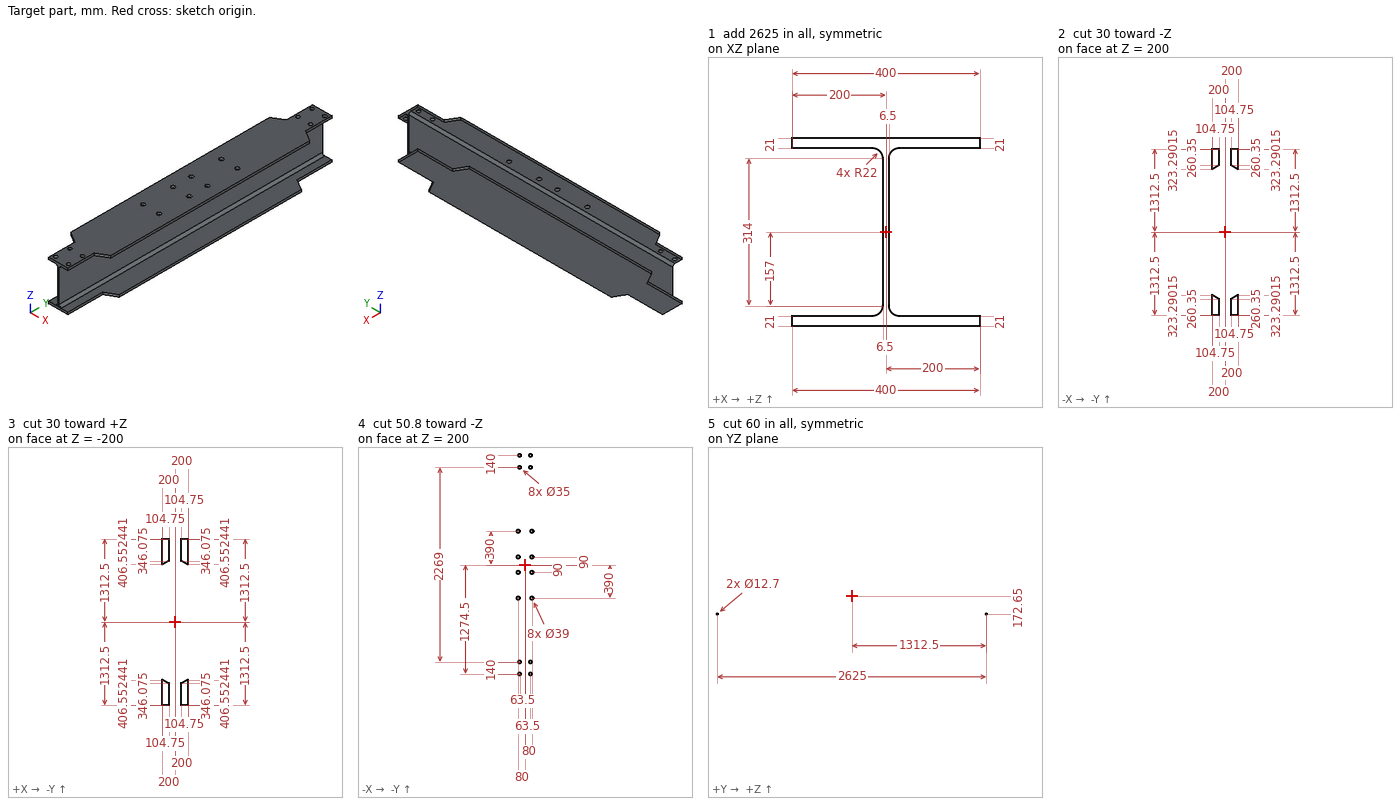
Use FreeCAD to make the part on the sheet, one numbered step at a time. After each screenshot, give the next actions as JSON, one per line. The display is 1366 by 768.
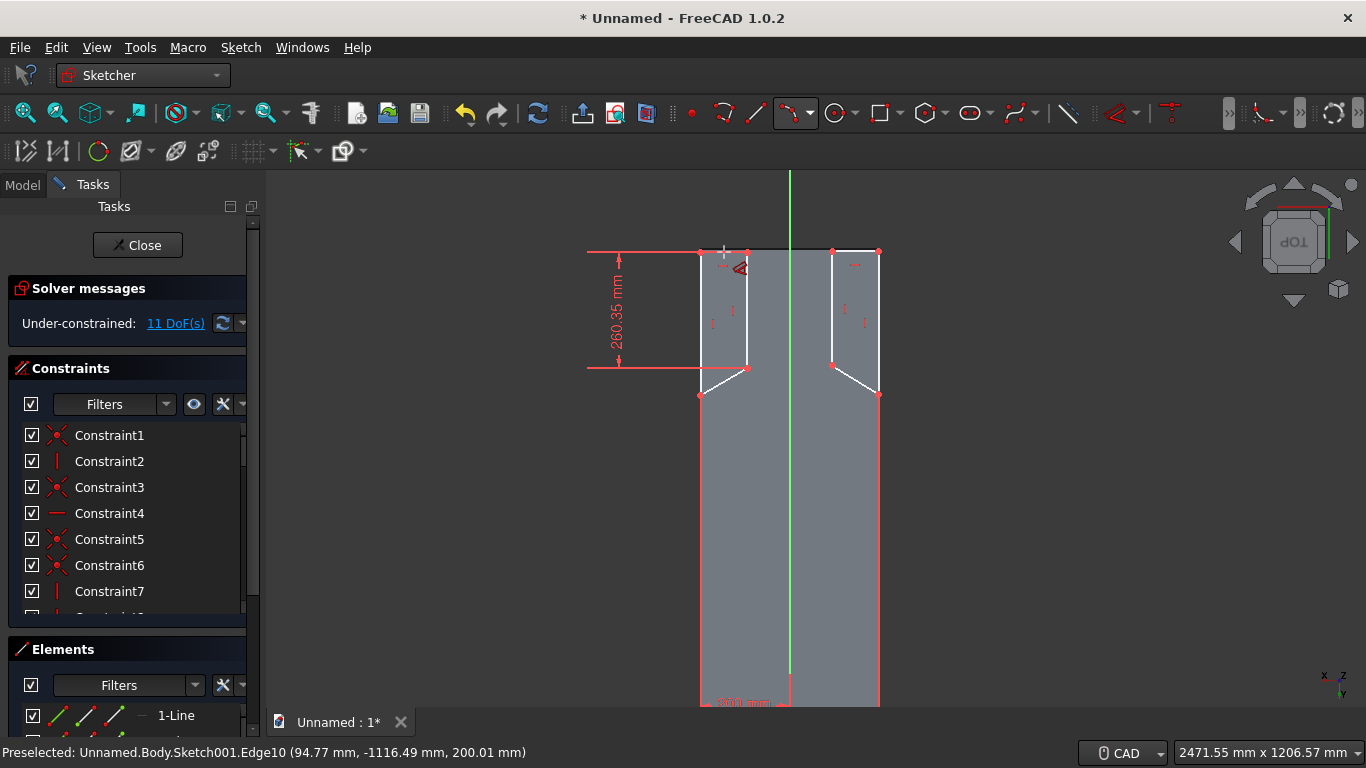
{"action": "left_click", "coordinate": [724, 252]}
{"action": "left_click", "coordinate": [724, 218]}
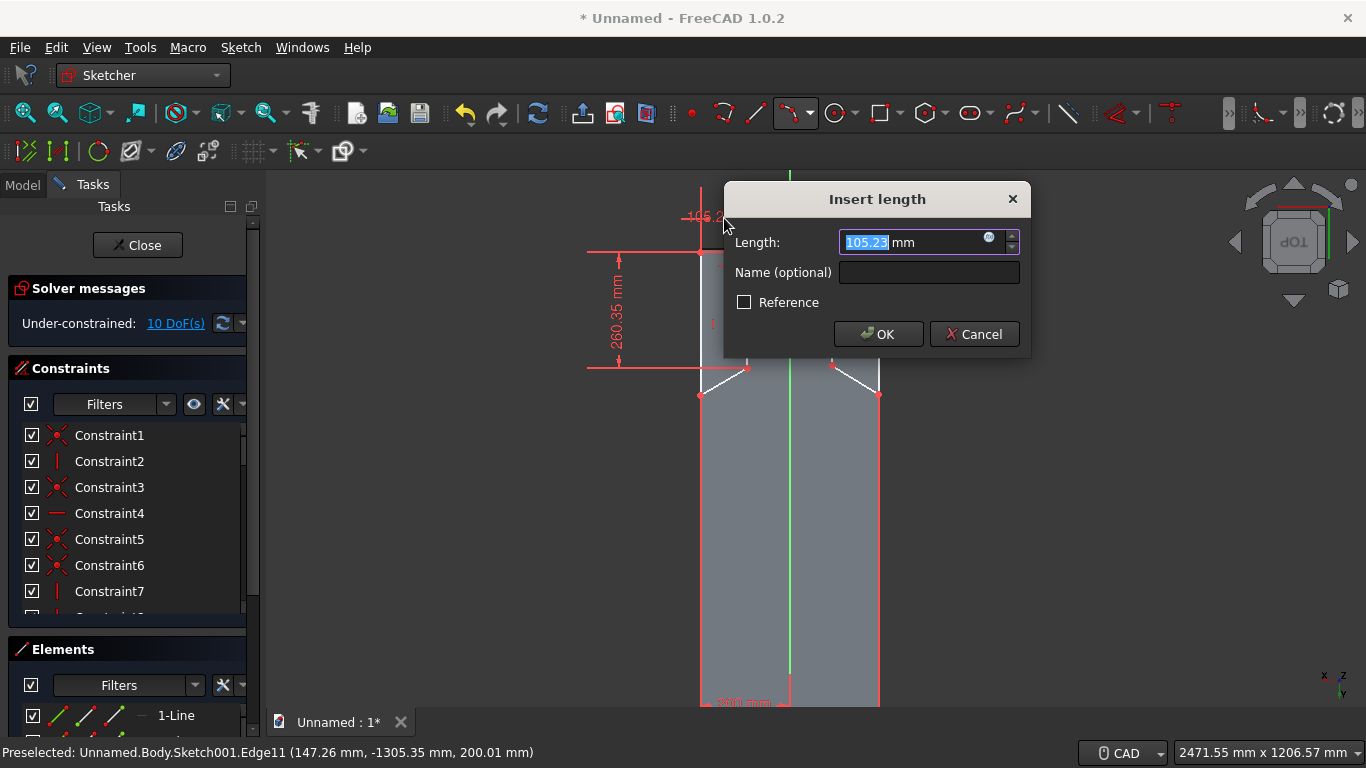
{"action": "type", "text": "104.75"}
{"action": "key", "text": "Return"}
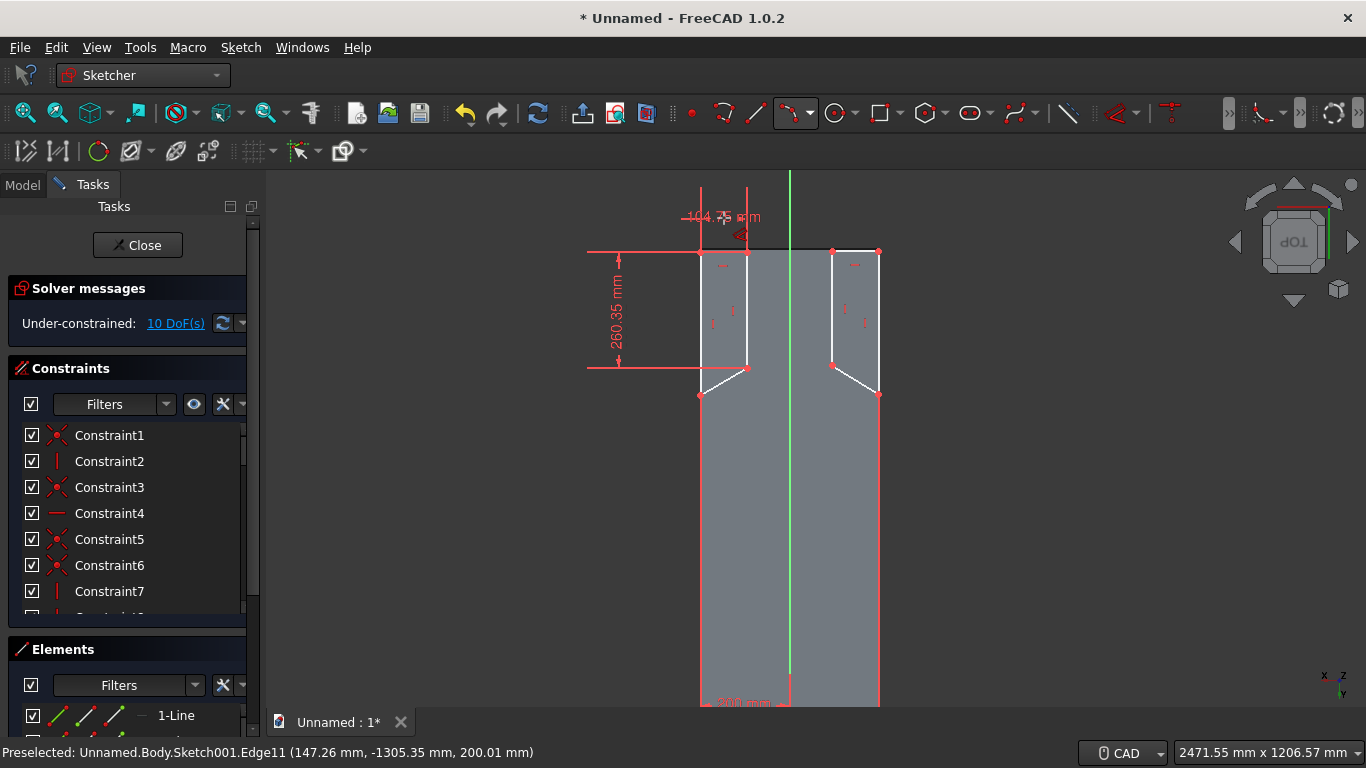
{"action": "left_click", "coordinate": [865, 251]}
{"action": "left_click", "coordinate": [855, 217]}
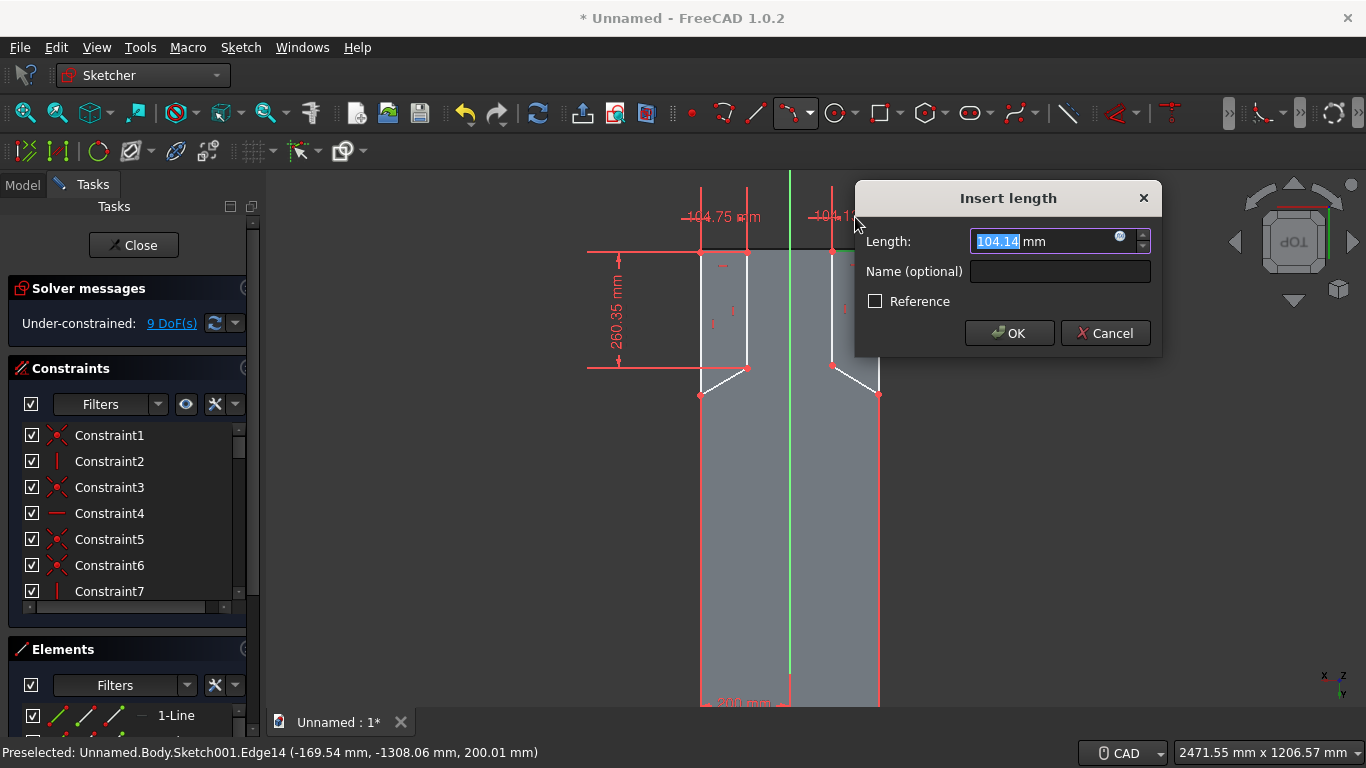
{"action": "type", "text": "104.75"}
{"action": "key", "text": "Return"}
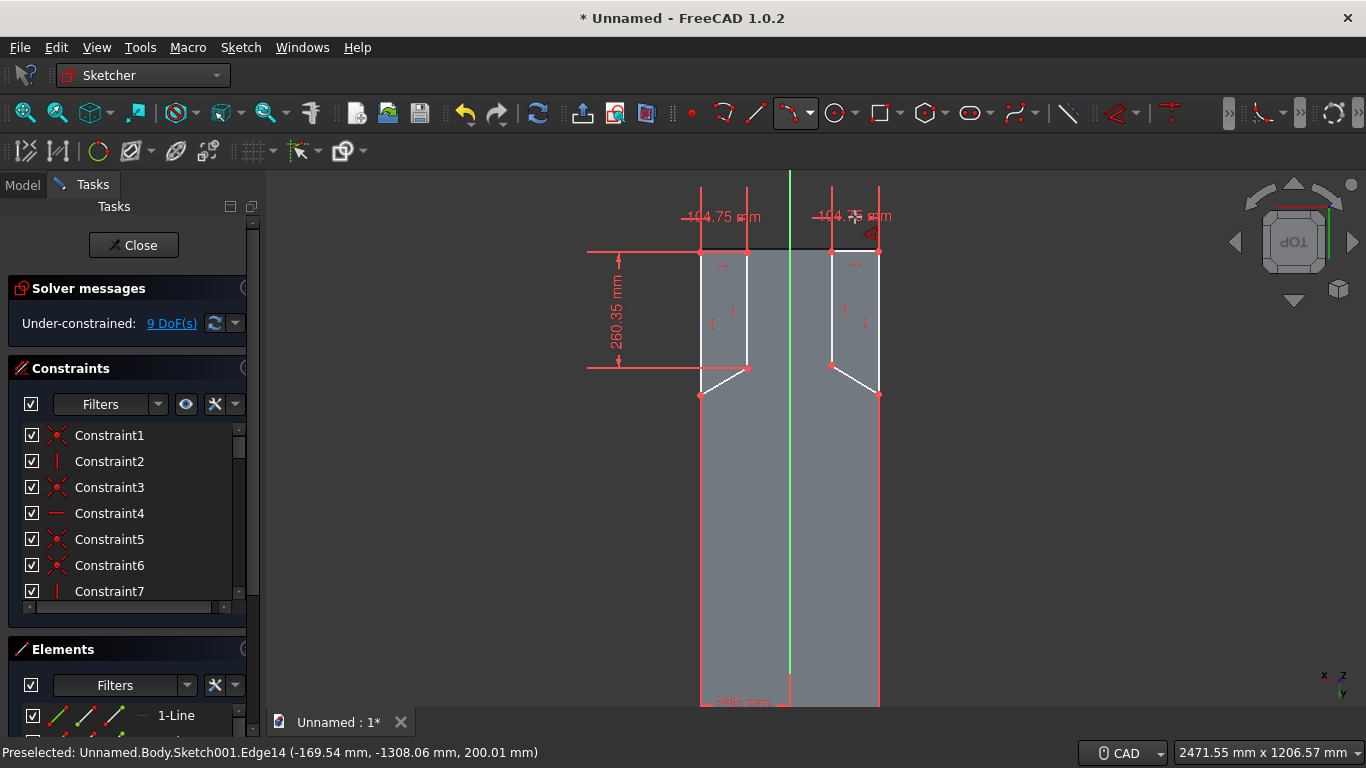
{"action": "left_click", "coordinate": [832, 286]}
{"action": "left_click", "coordinate": [774, 309]}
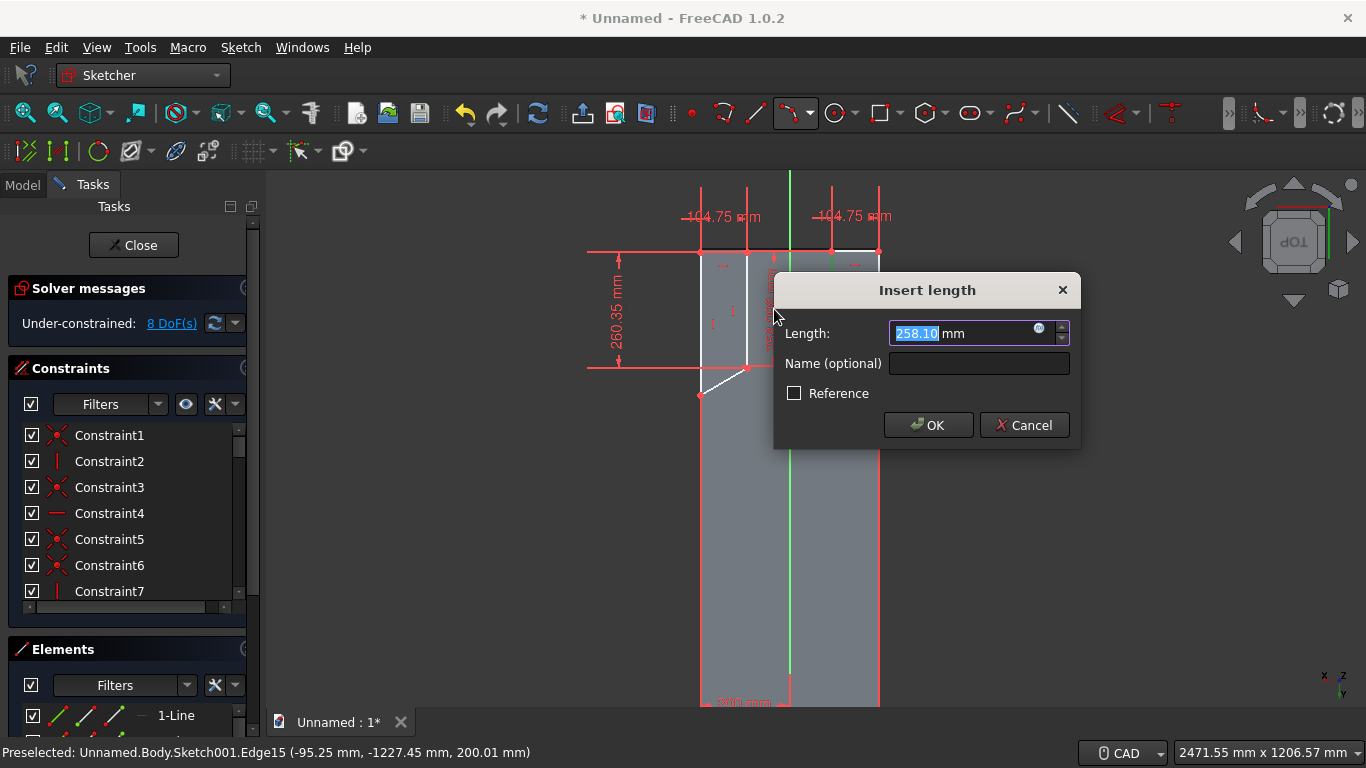
{"action": "type", "text": "260.35"}
{"action": "key", "text": "Return"}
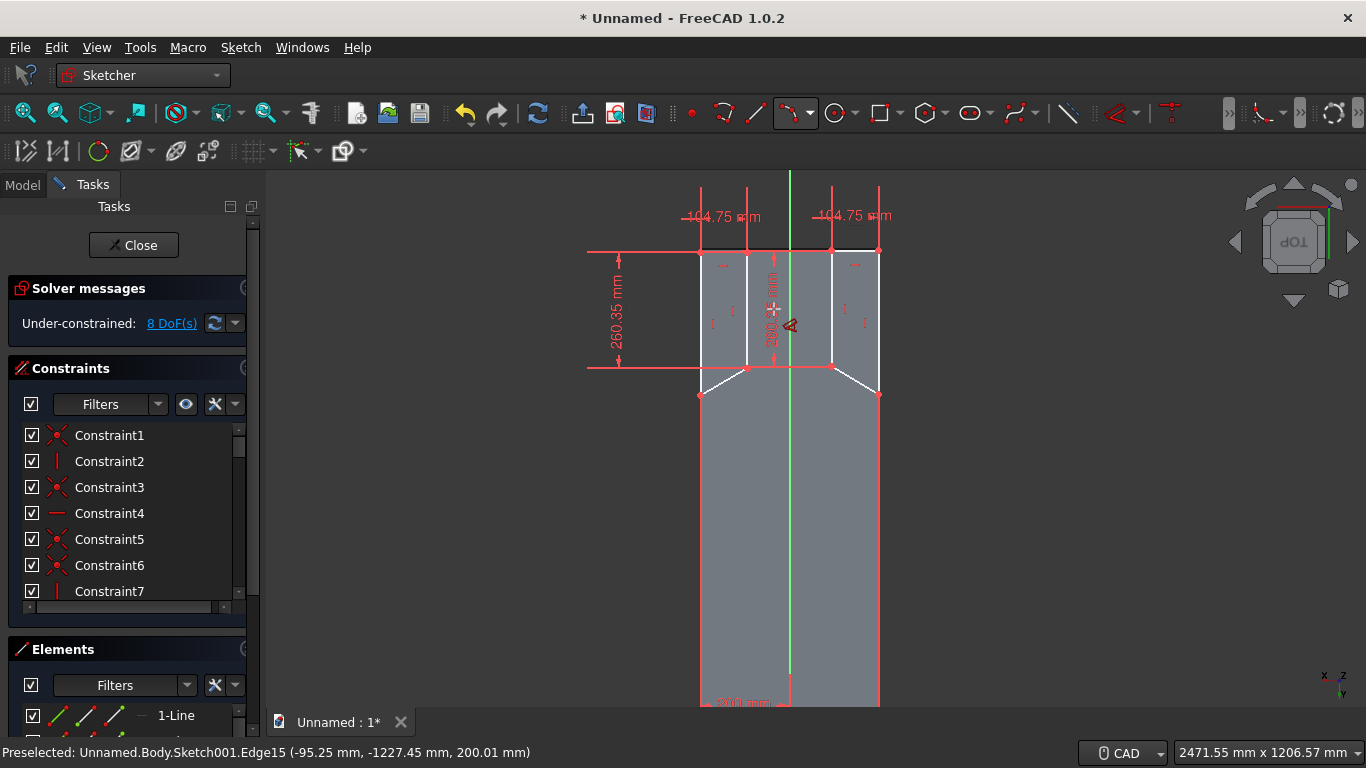
{"action": "scroll", "coordinate": [729, 268], "scroll_direction": "down", "scroll_amount": 6}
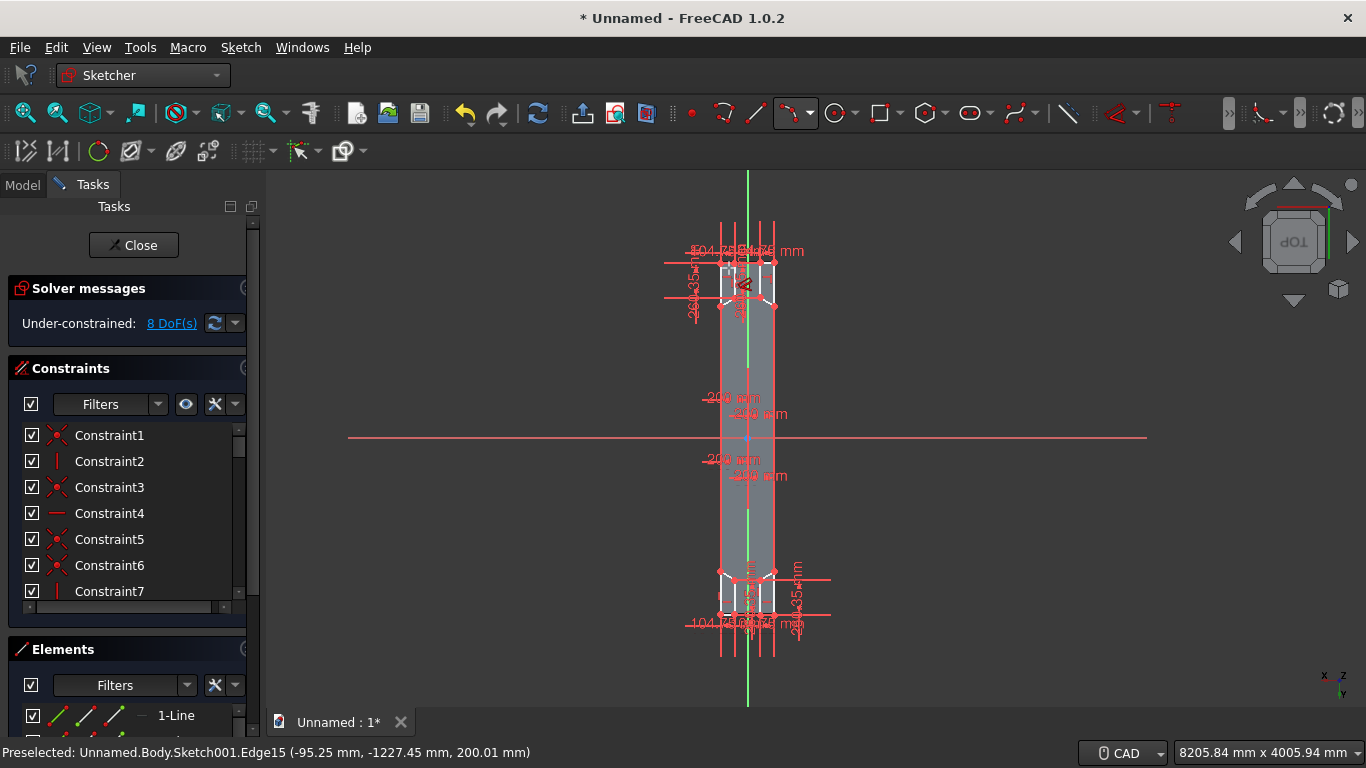
{"action": "left_click", "coordinate": [760, 615]}
{"action": "left_click", "coordinate": [794, 527]}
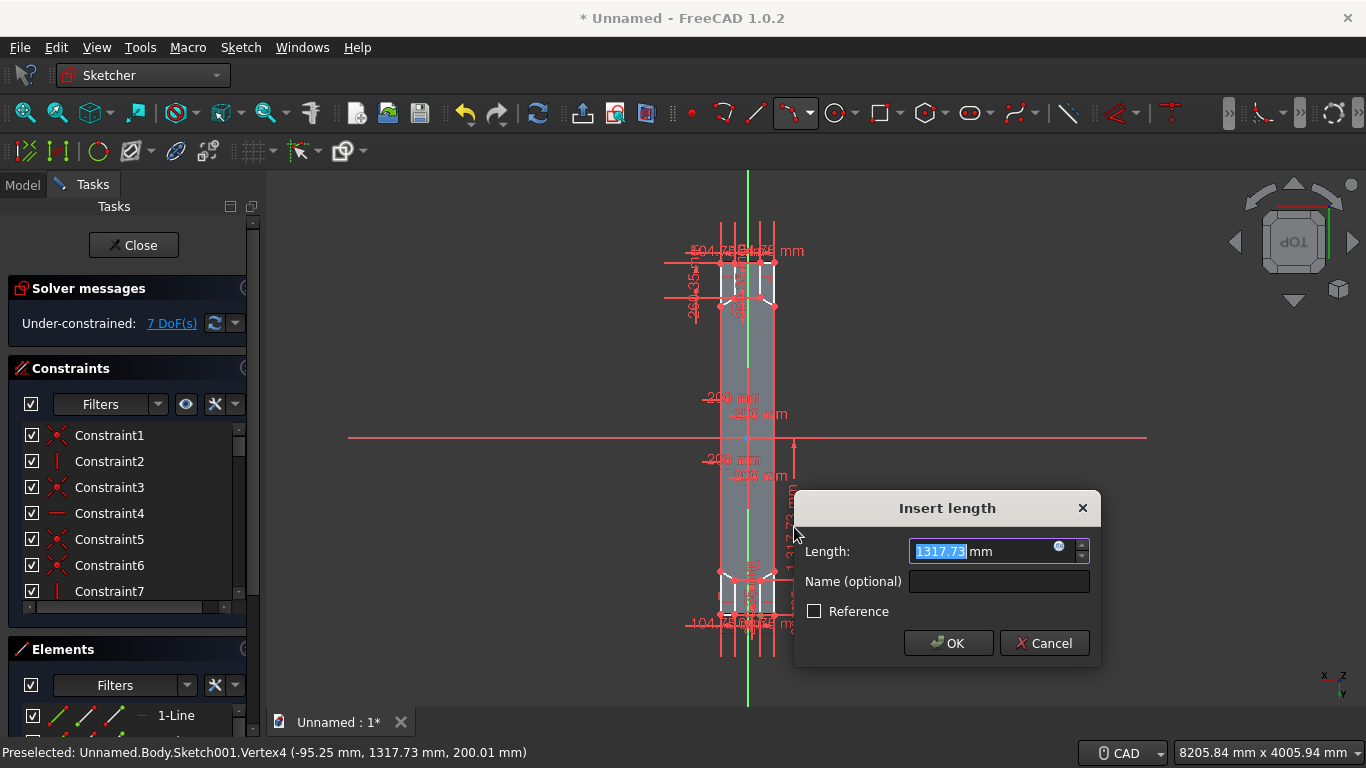
{"action": "type", "text": "1312.5"}
{"action": "key", "text": "Return"}